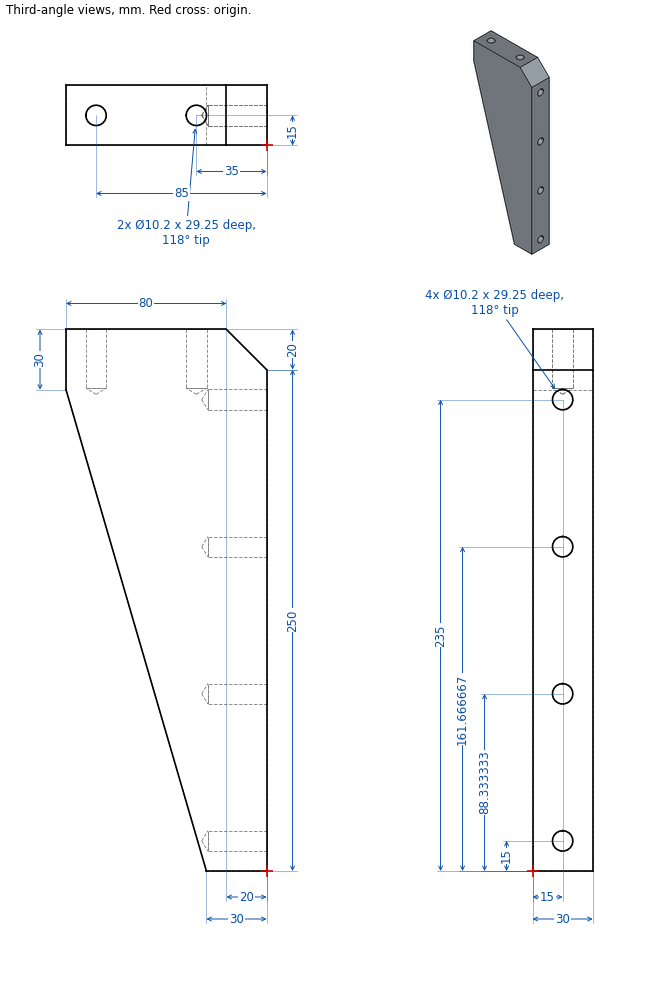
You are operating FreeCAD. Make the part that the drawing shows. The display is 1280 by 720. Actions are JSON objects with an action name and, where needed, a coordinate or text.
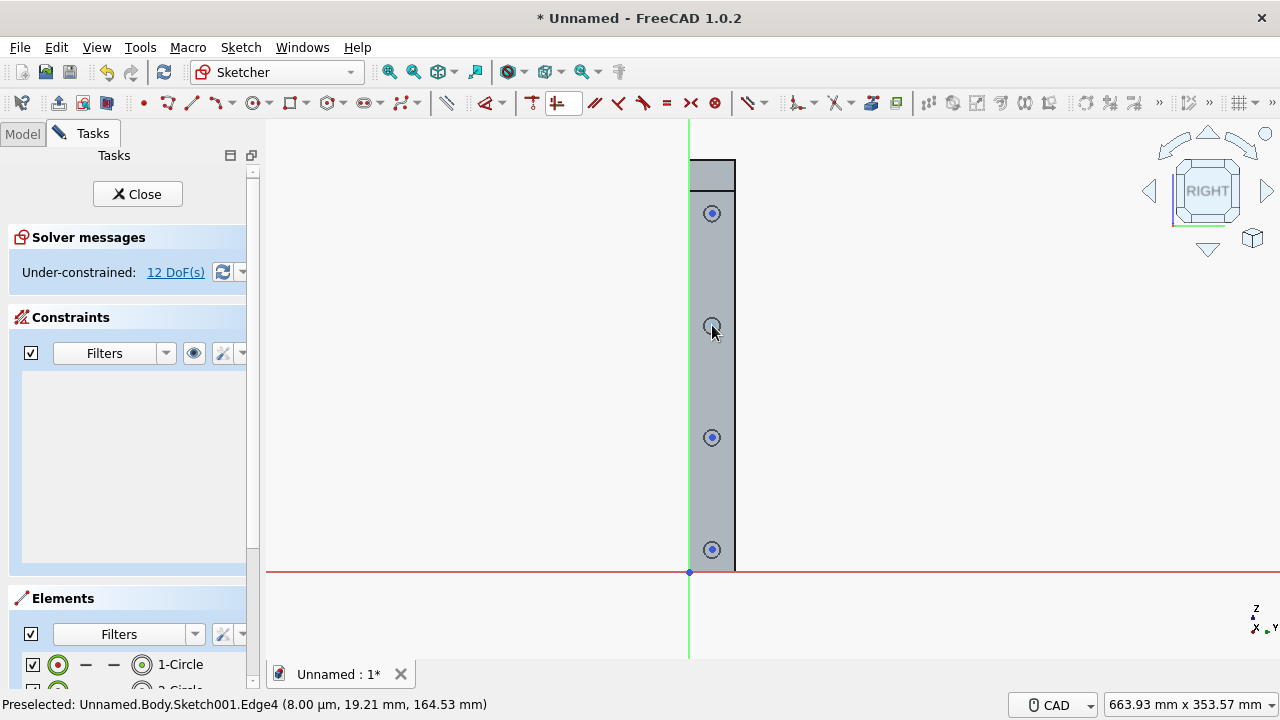
{"action": "scroll", "coordinate": [718, 208], "scroll_direction": "up", "scroll_amount": 3}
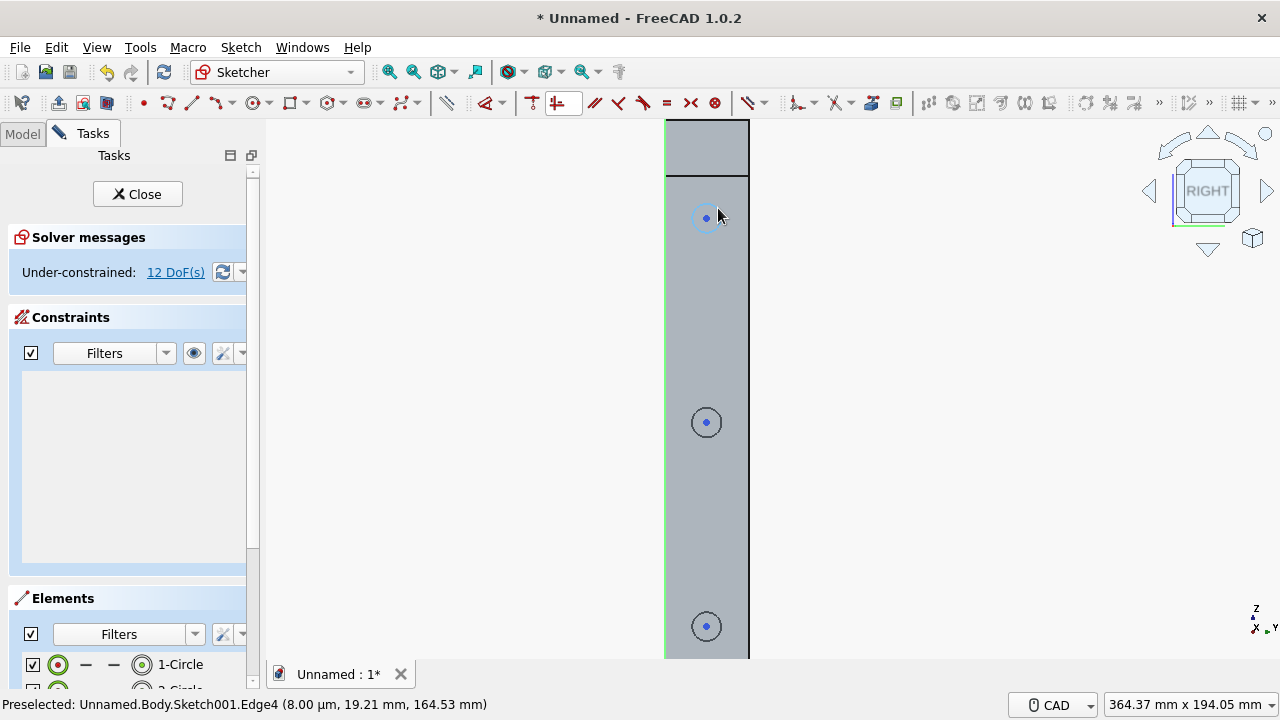
{"action": "left_click", "coordinate": [717, 208]}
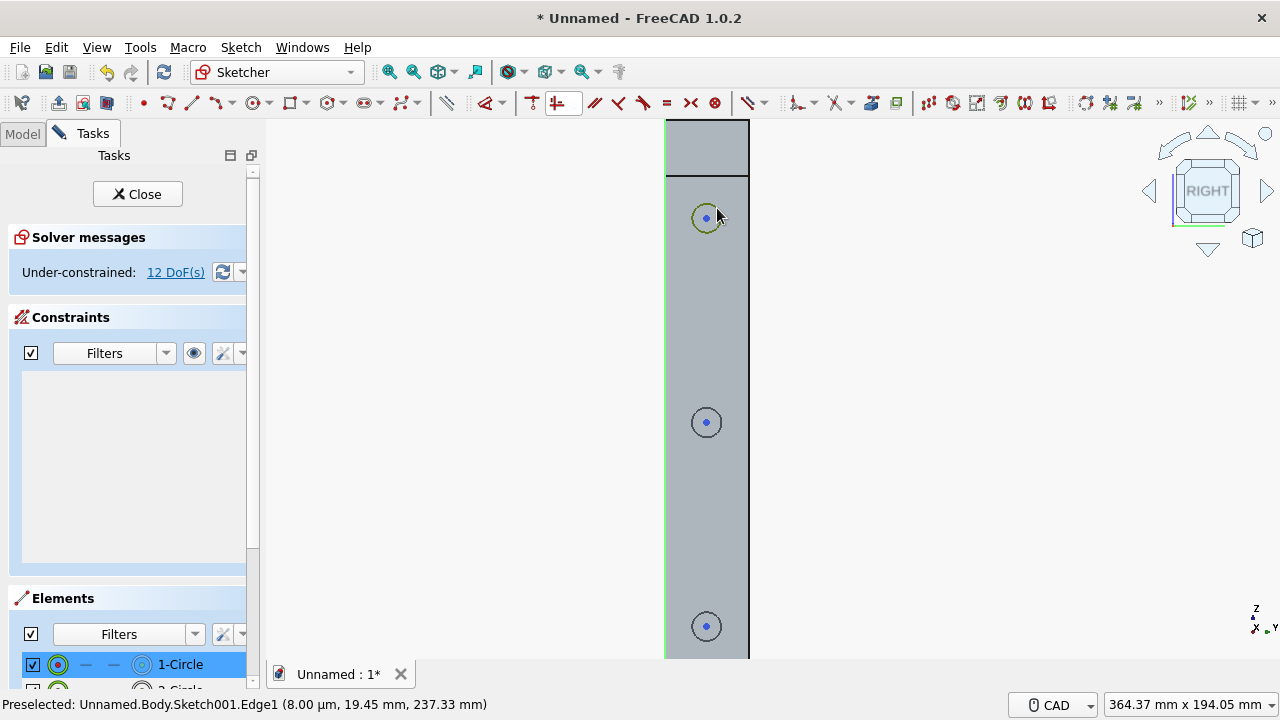
{"action": "scroll", "coordinate": [718, 208], "scroll_direction": "down", "scroll_amount": 3}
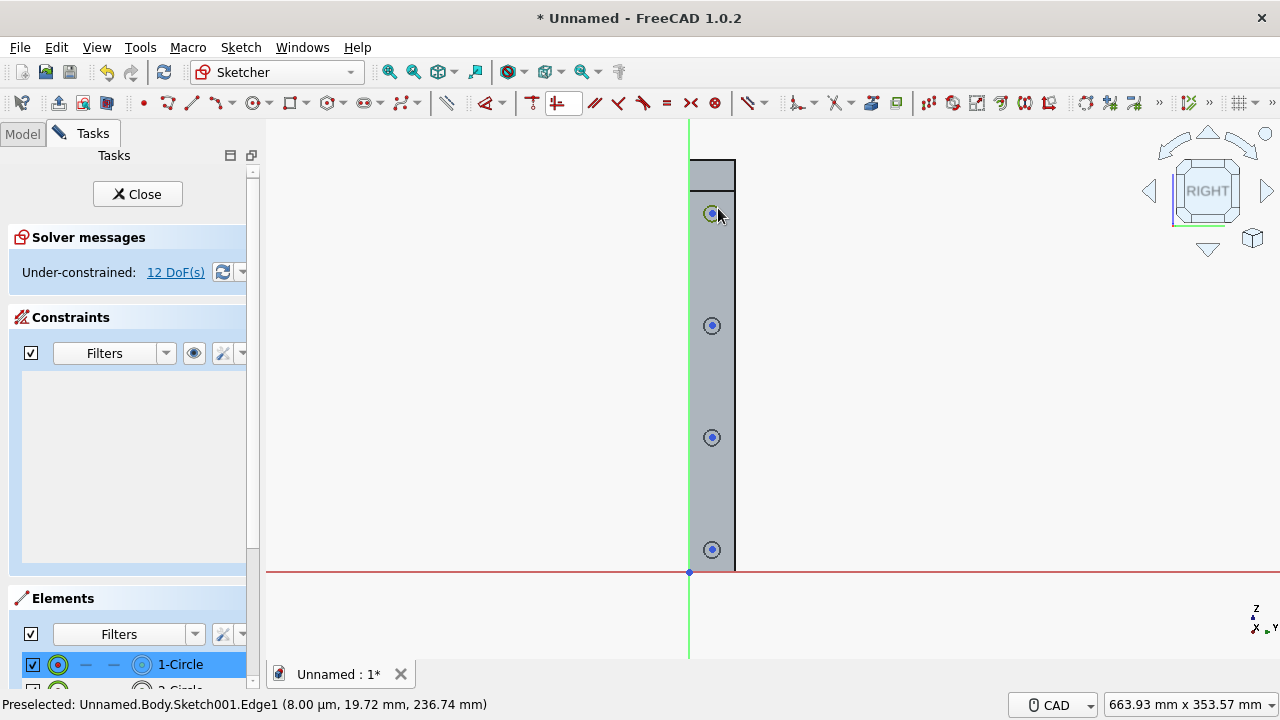
{"action": "scroll", "coordinate": [718, 544], "scroll_direction": "up", "scroll_amount": 3}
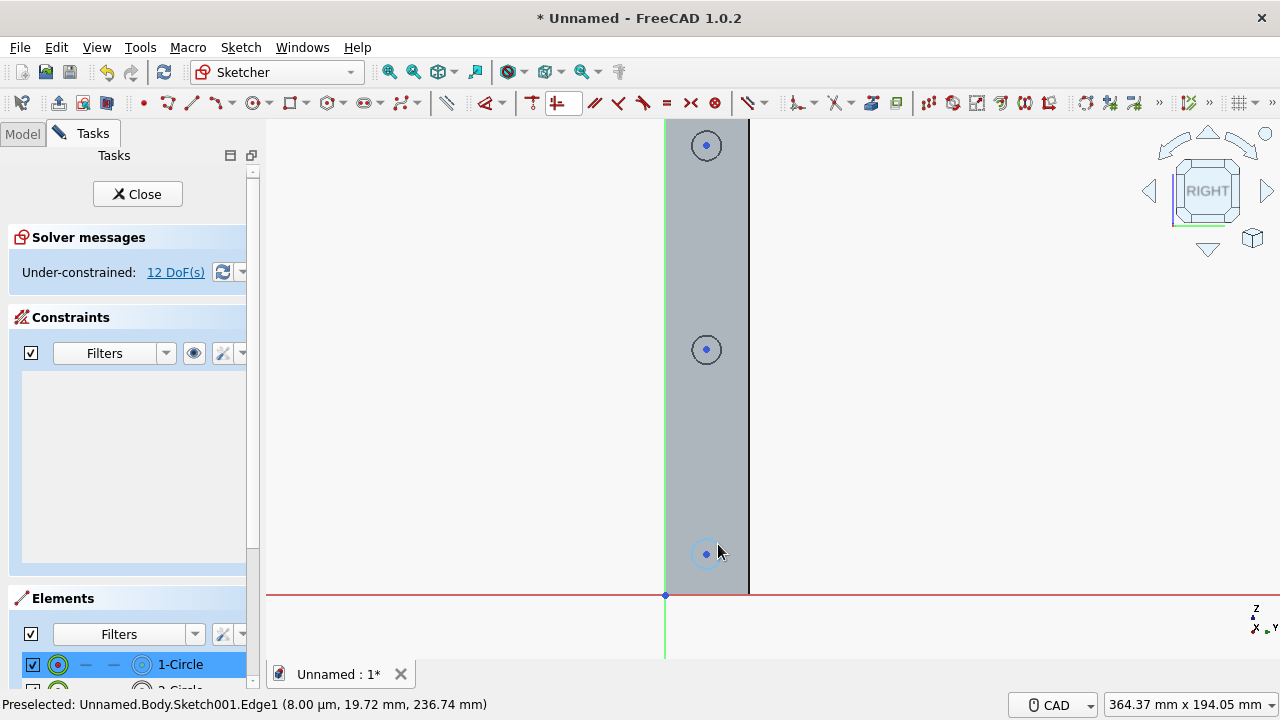
{"action": "left_click", "coordinate": [717, 544]}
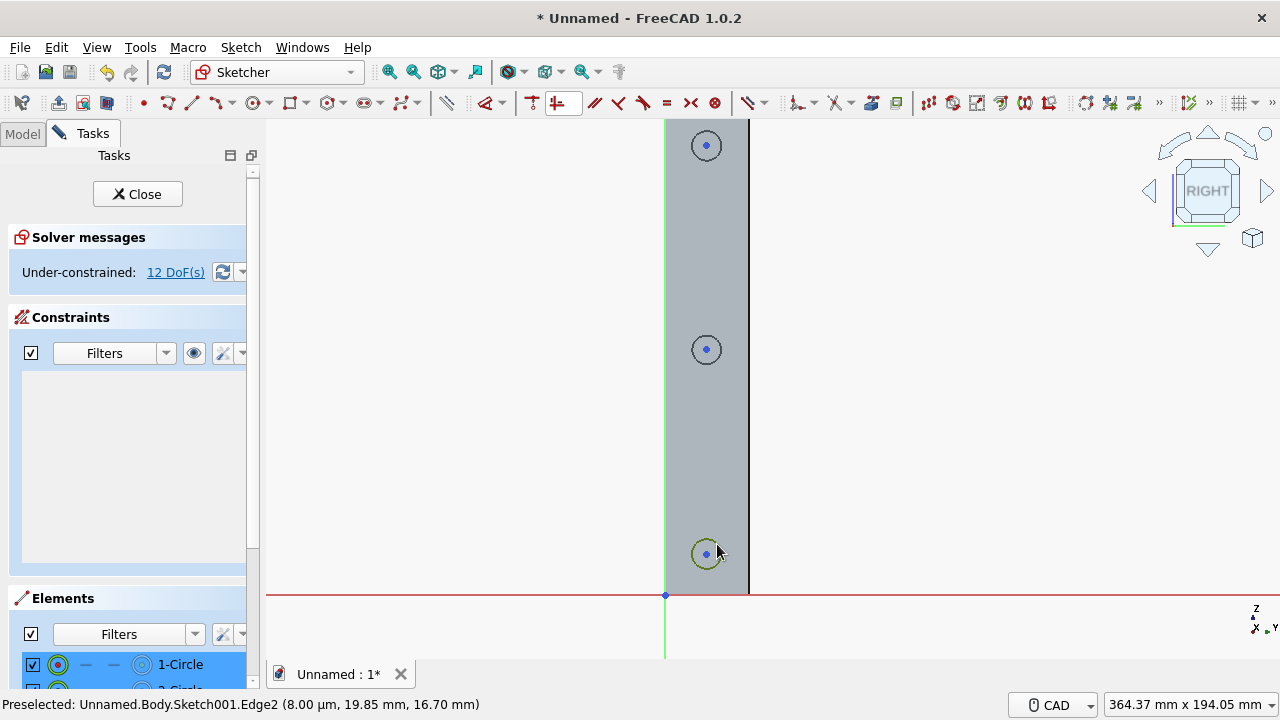
{"action": "left_click", "coordinate": [717, 340]}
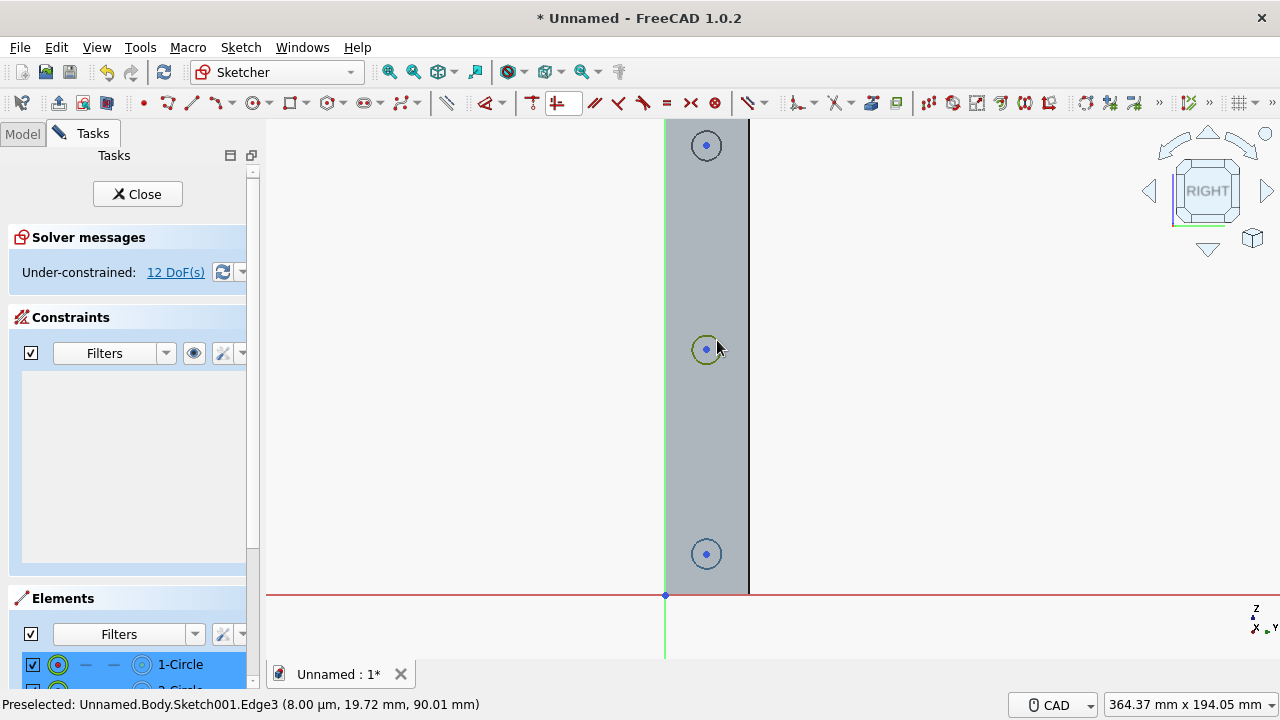
{"action": "left_click", "coordinate": [696, 156]}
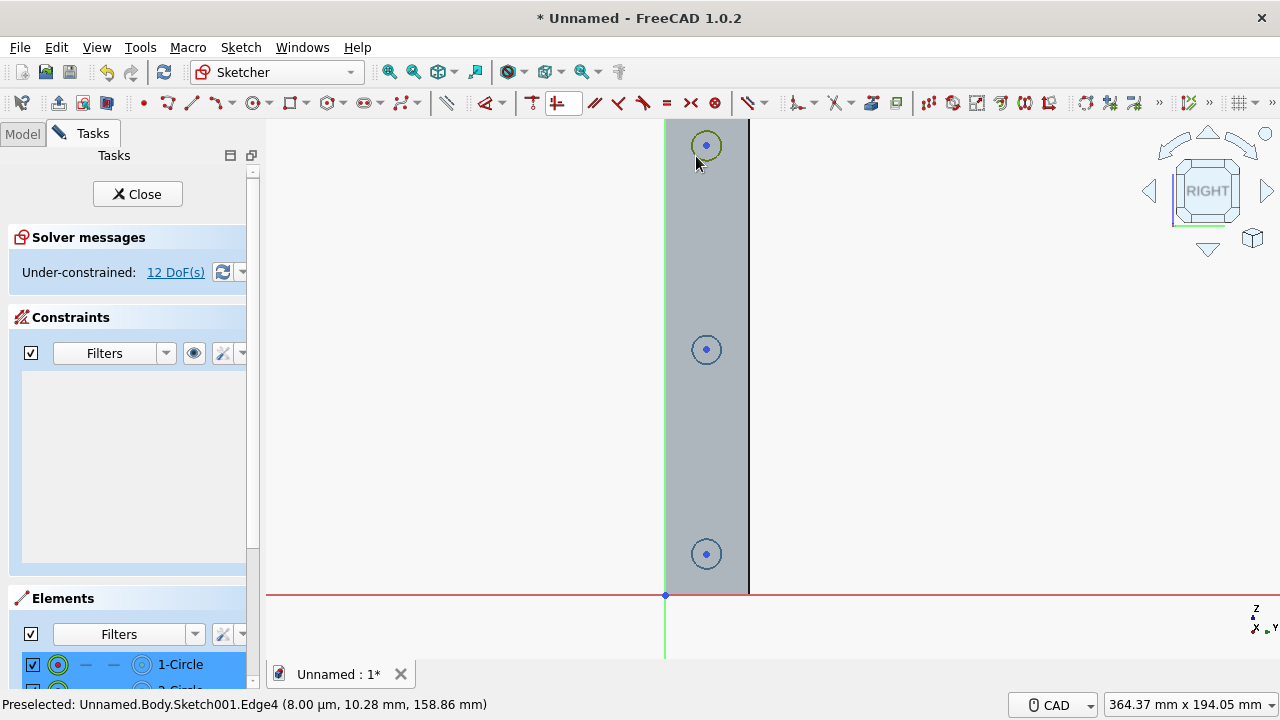
{"action": "key", "text": "e"}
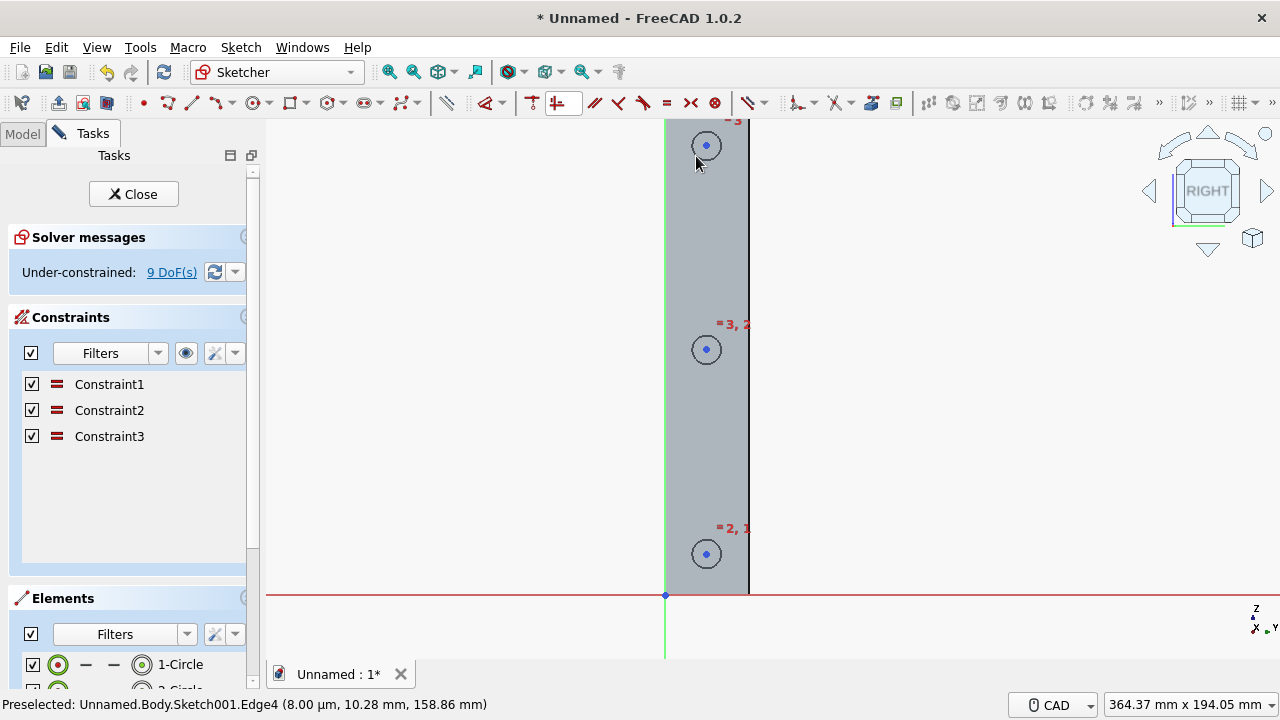
{"action": "left_click", "coordinate": [486, 104]}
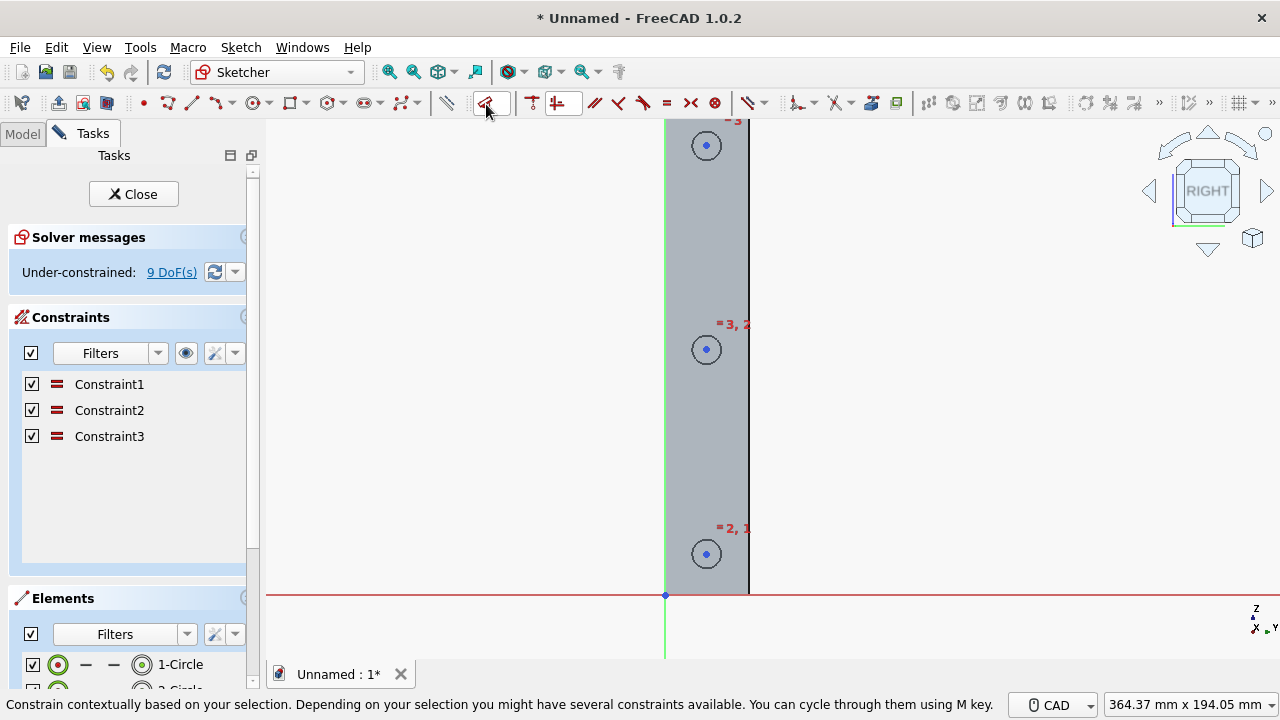
{"action": "scroll", "coordinate": [718, 545], "scroll_direction": "down", "scroll_amount": 3}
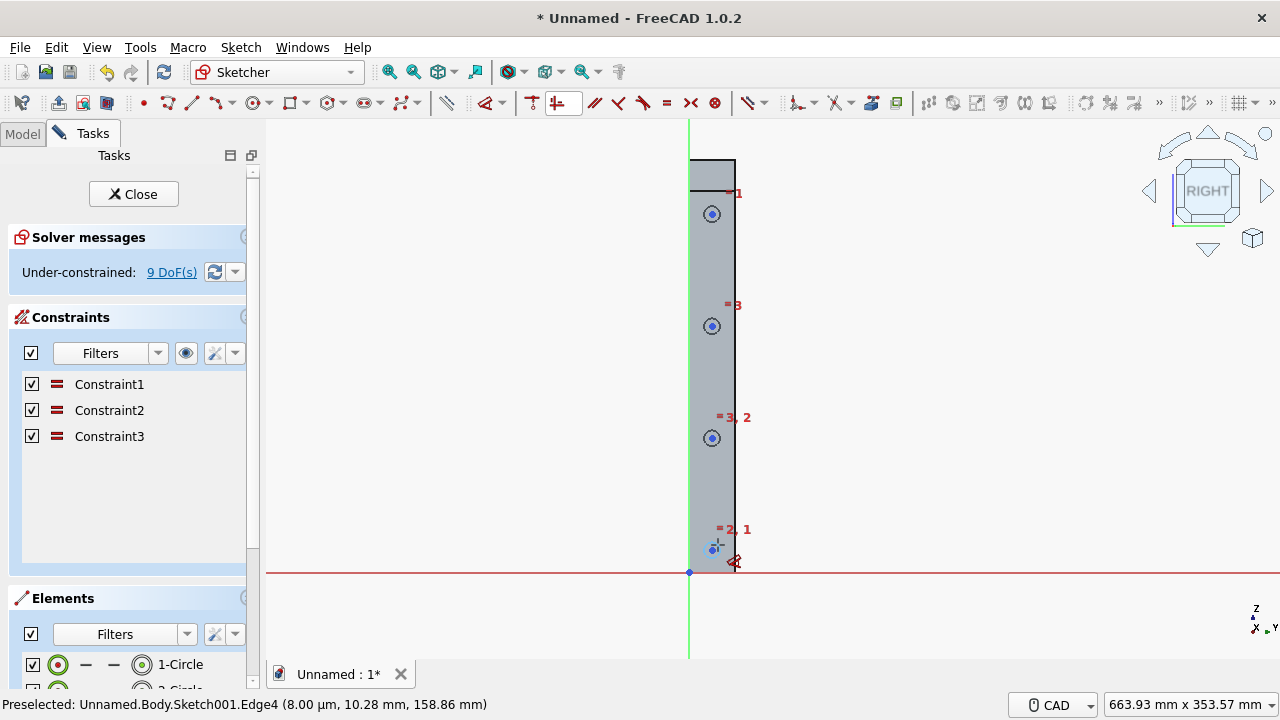
{"action": "scroll", "coordinate": [718, 209], "scroll_direction": "up", "scroll_amount": 5}